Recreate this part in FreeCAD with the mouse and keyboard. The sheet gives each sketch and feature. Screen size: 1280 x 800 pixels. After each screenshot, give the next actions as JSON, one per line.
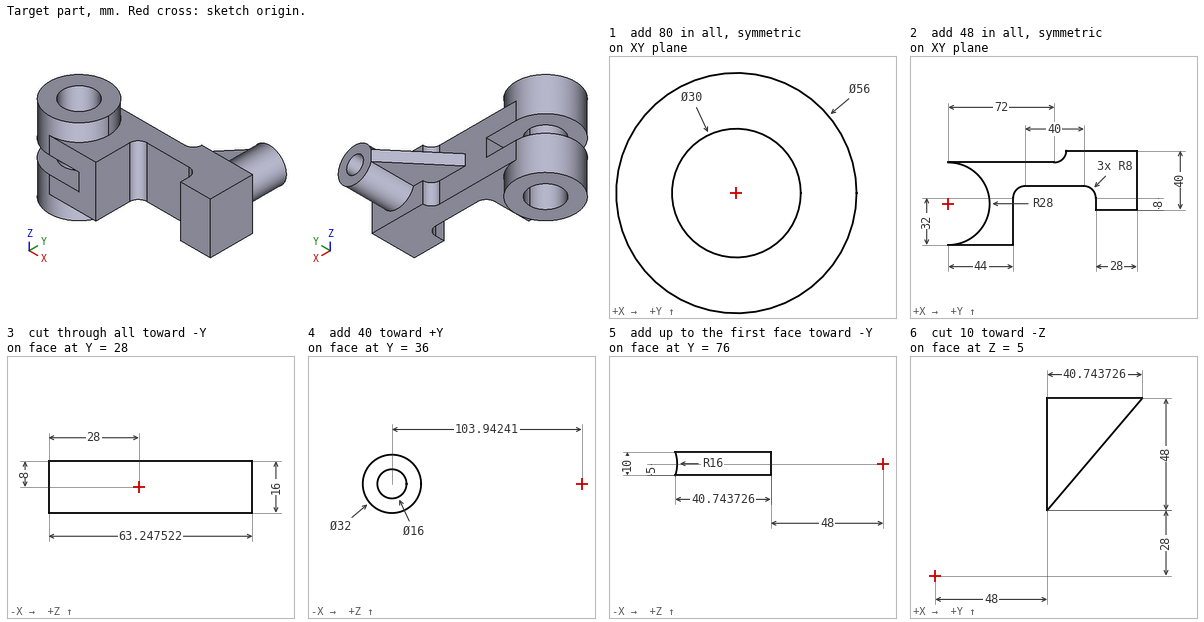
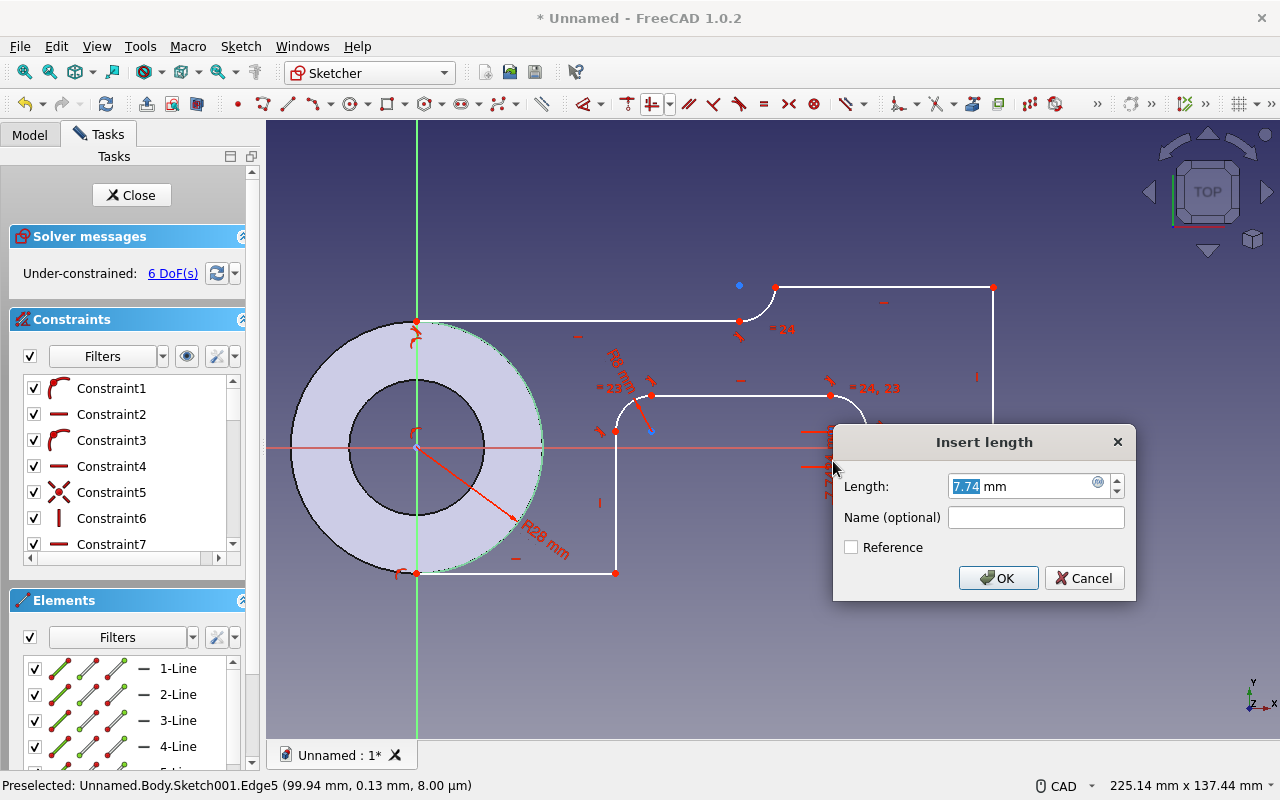
{"action": "type", "text": "8"}
{"action": "key", "text": "Return"}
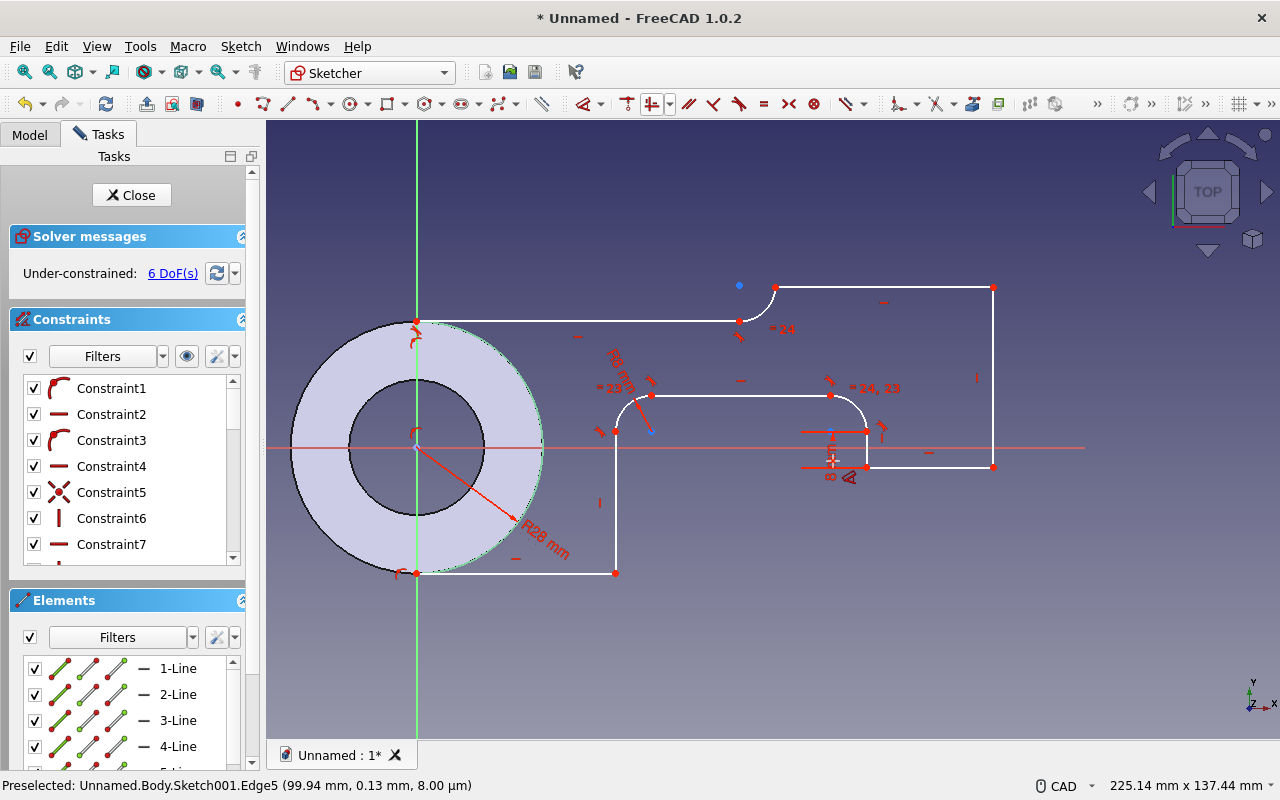
{"action": "left_click", "coordinate": [643, 321]}
{"action": "left_click", "coordinate": [578, 287]}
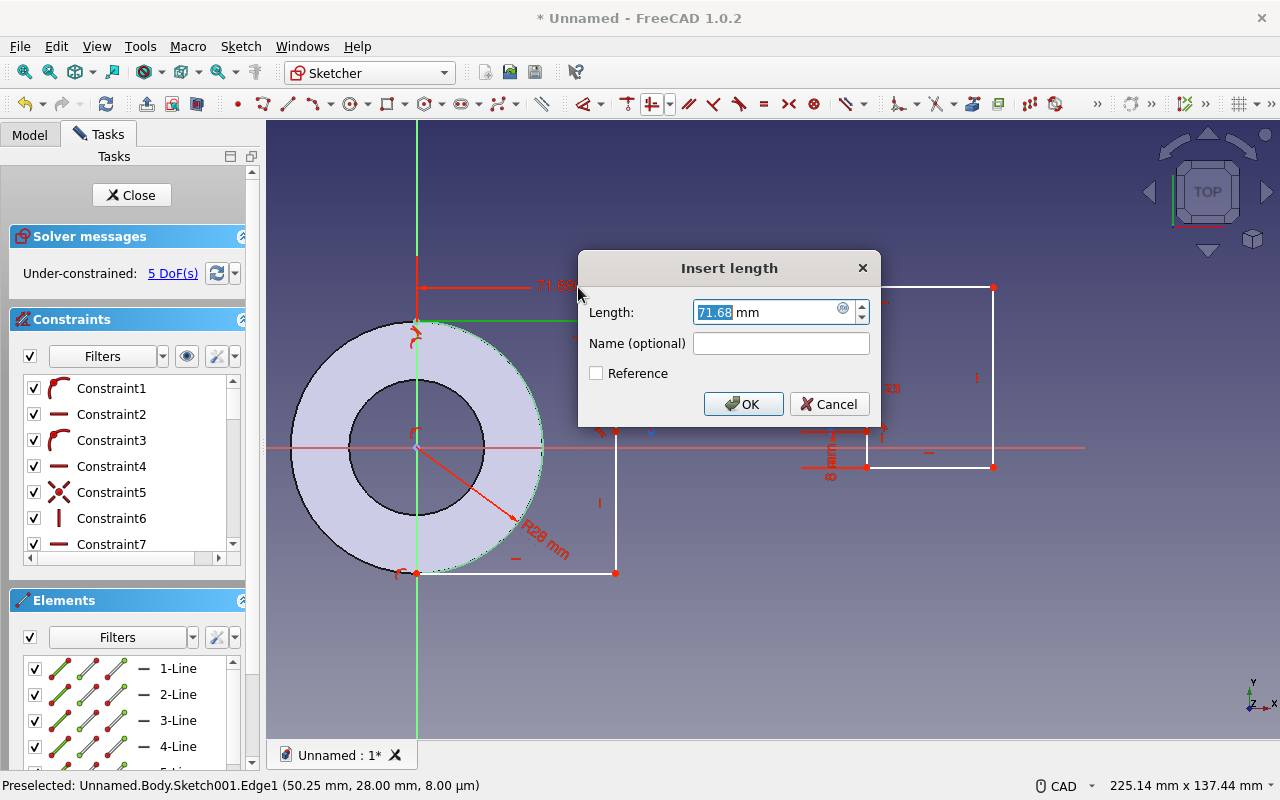
{"action": "type", "text": "72"}
{"action": "key", "text": "Return"}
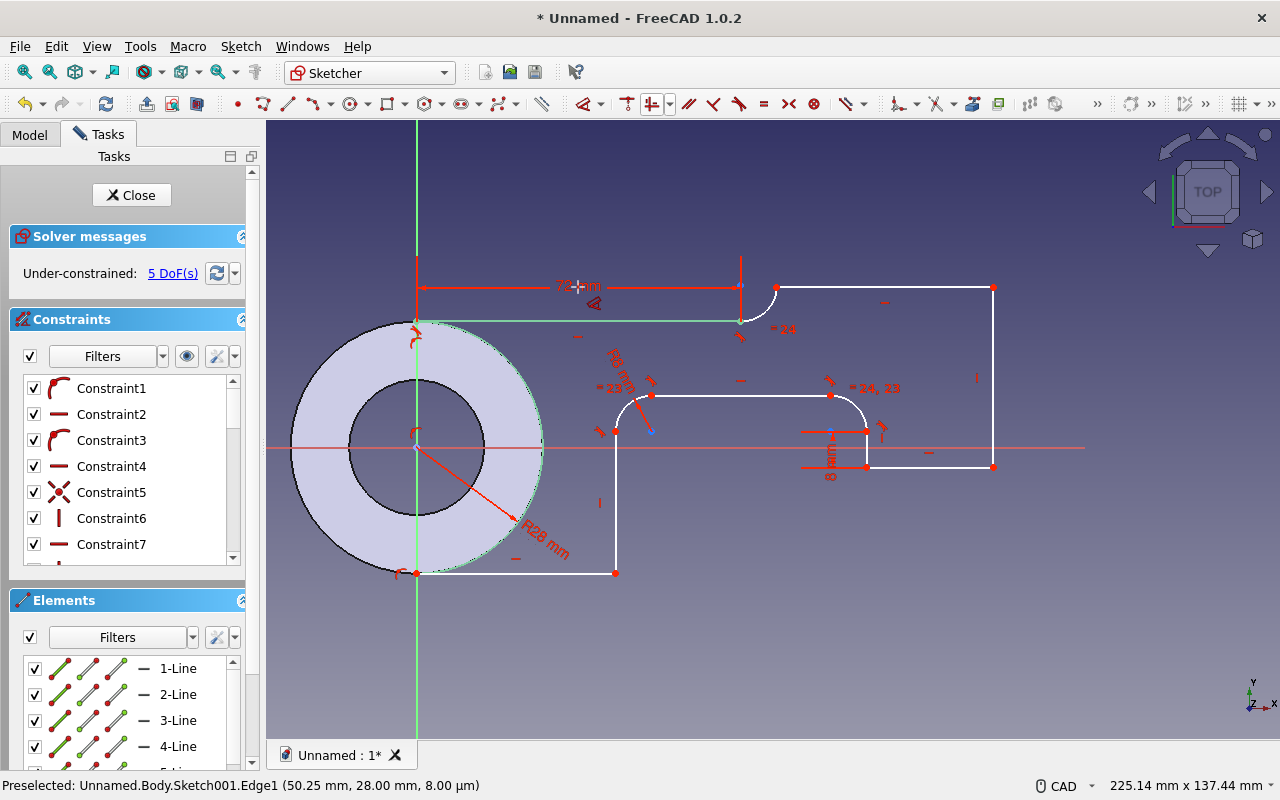
{"action": "left_click", "coordinate": [476, 574]}
{"action": "left_click", "coordinate": [516, 608]}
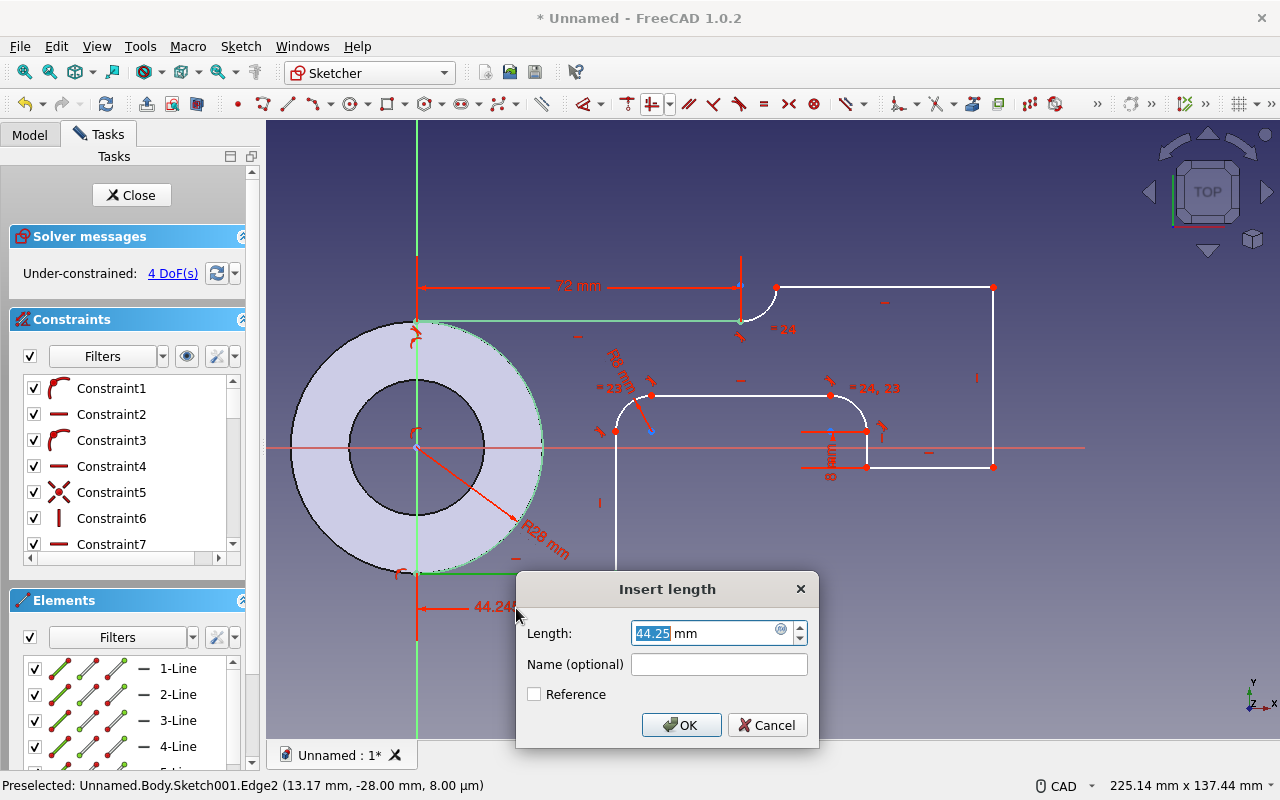
{"action": "type", "text": "44"}
{"action": "key", "text": "Return"}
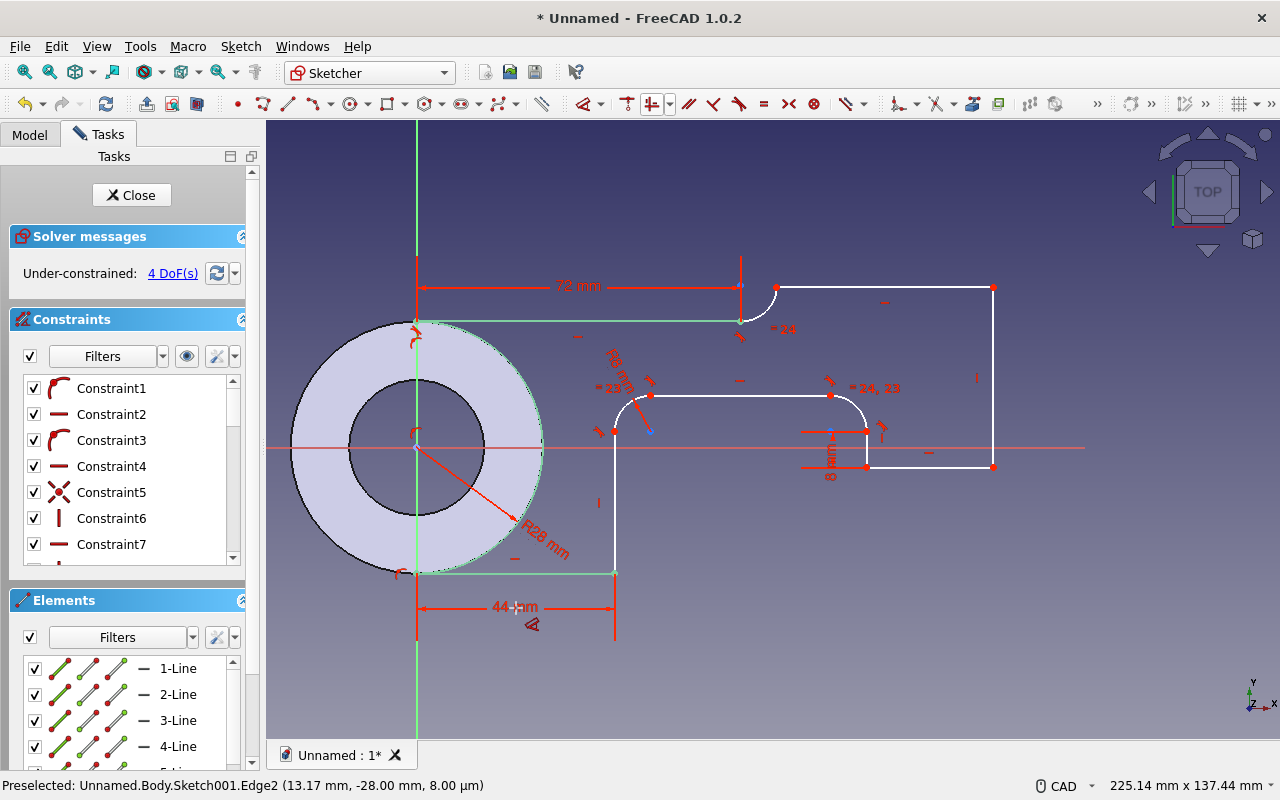
{"action": "left_click", "coordinate": [615, 531]}
{"action": "left_click", "coordinate": [581, 503]}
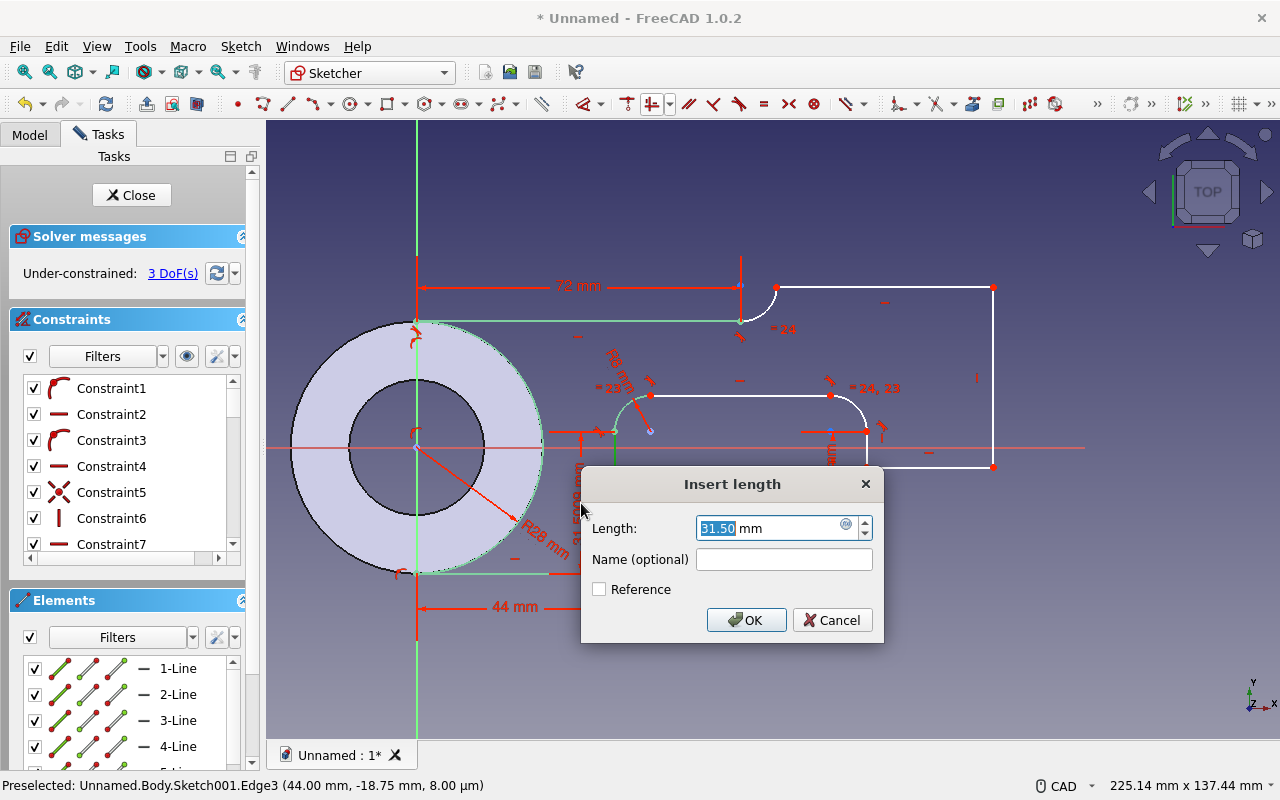
{"action": "type", "text": "32"}
{"action": "key", "text": "Return"}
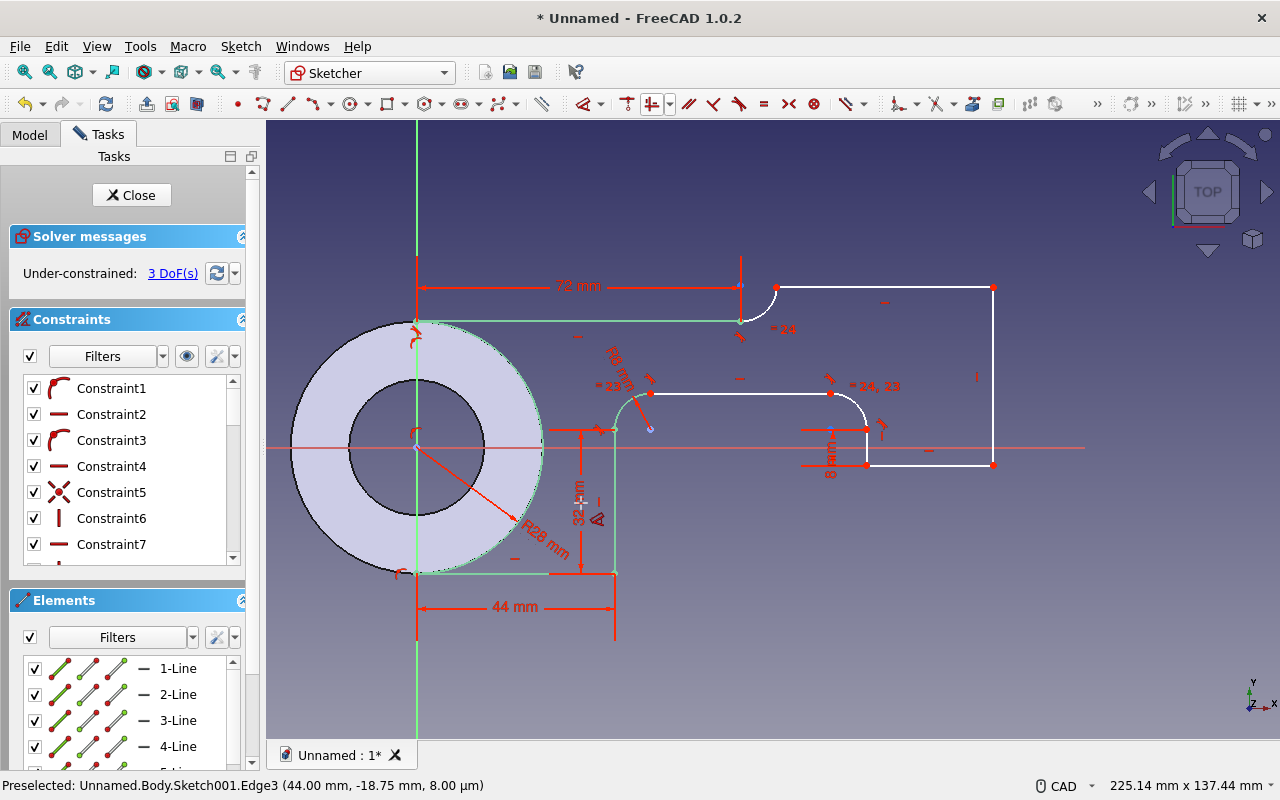
{"action": "left_click", "coordinate": [705, 394]}
{"action": "left_click", "coordinate": [741, 360]}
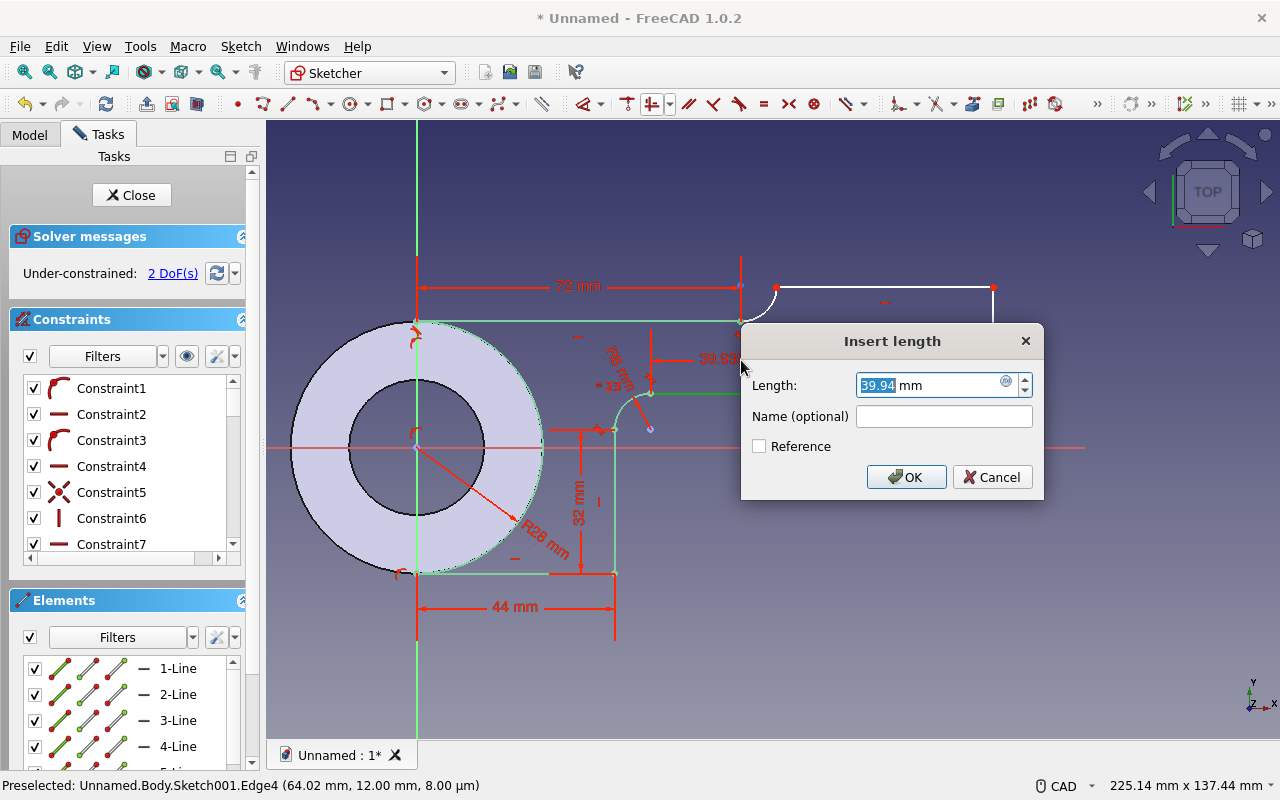
{"action": "type", "text": "40"}
{"action": "key", "text": "Return"}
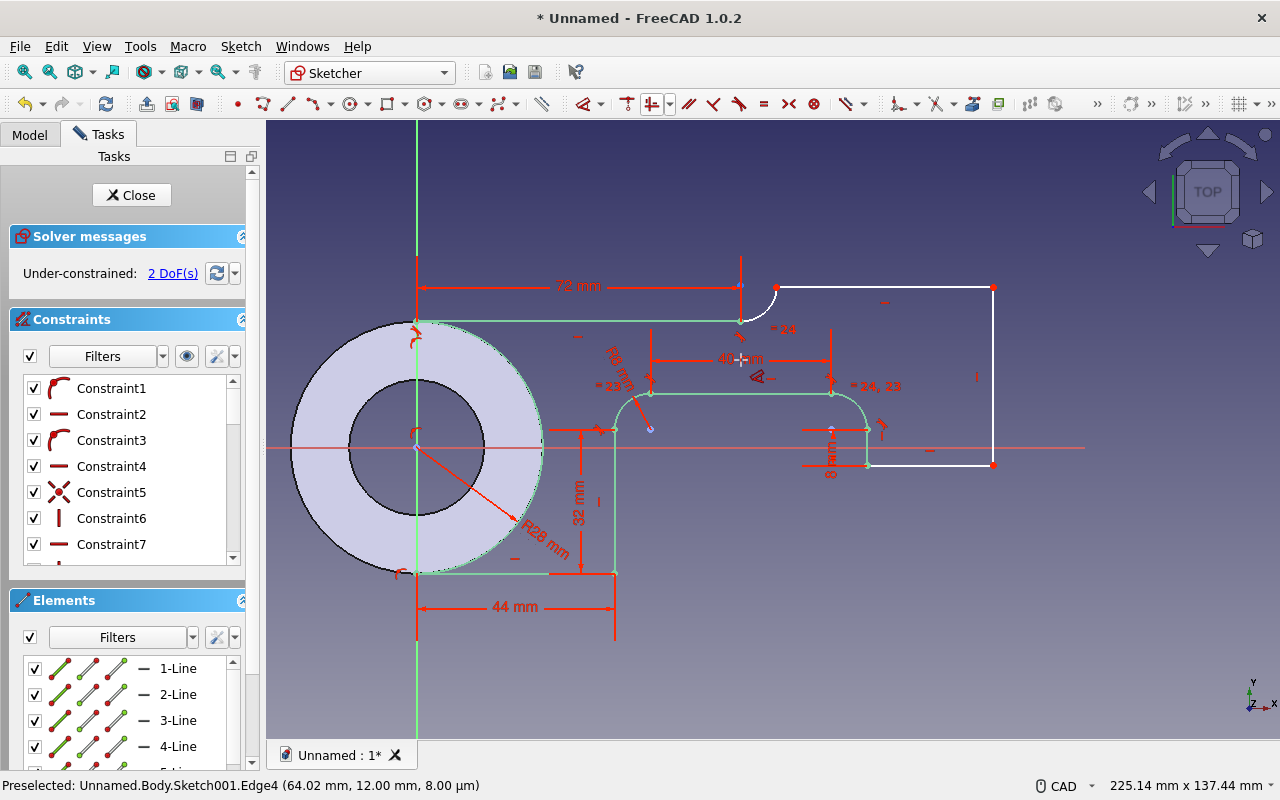
{"action": "left_click", "coordinate": [905, 466]}
{"action": "left_click", "coordinate": [930, 500]}